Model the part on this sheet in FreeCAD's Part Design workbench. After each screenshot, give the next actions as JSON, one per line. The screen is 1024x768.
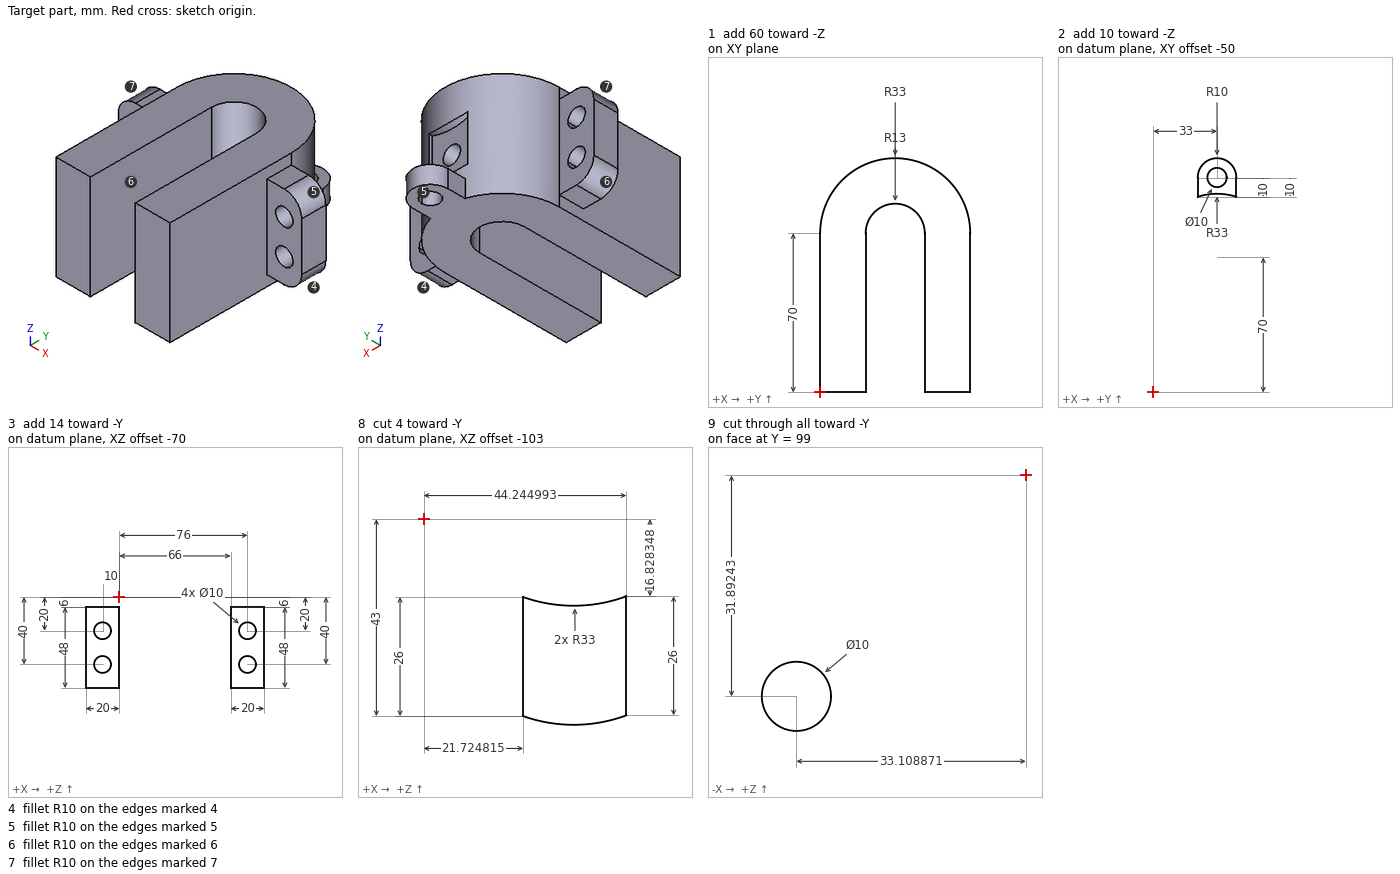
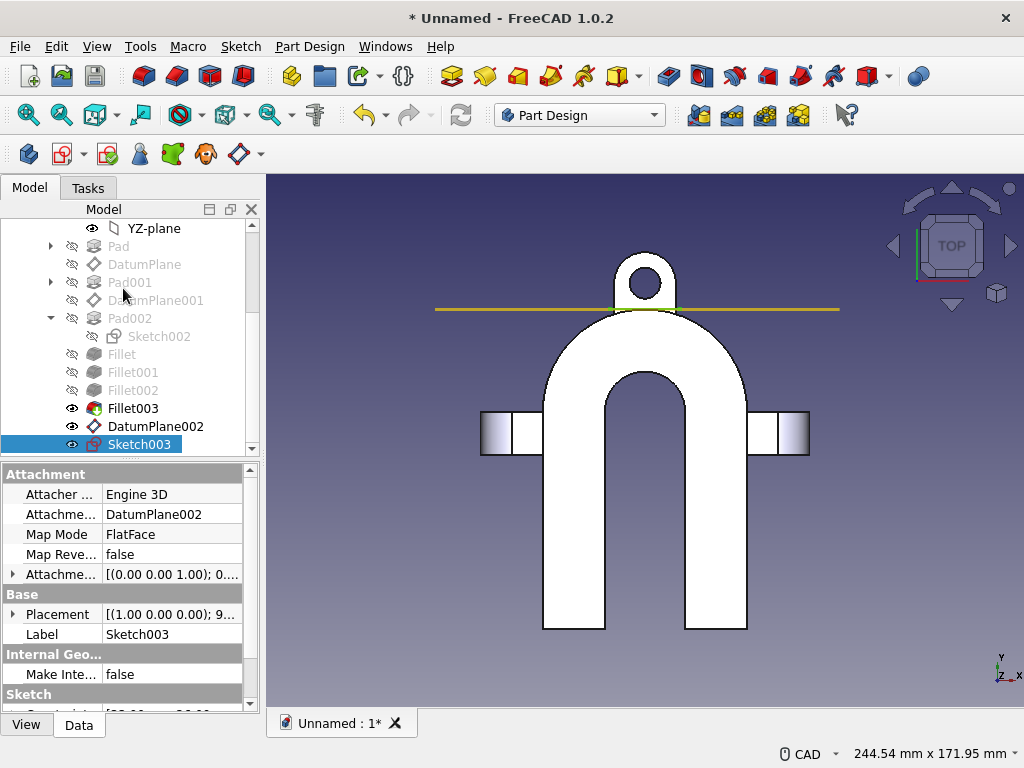
{"action": "left_click", "coordinate": [669, 76]}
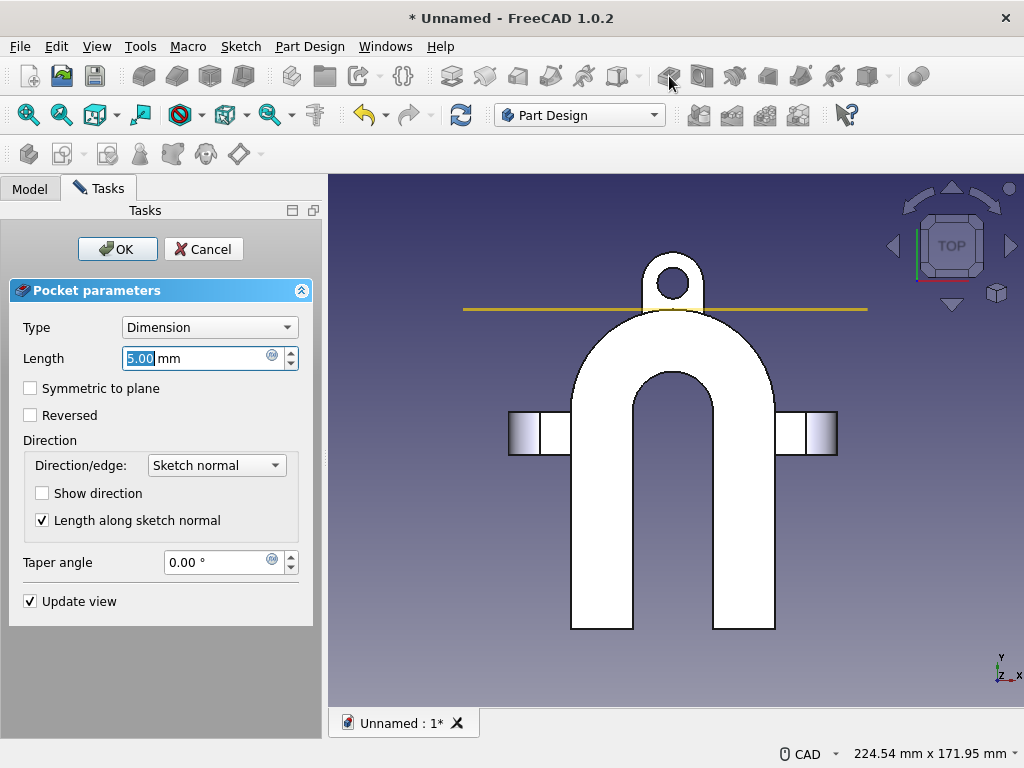
{"action": "type", "text": "4"}
{"action": "key", "text": "Tab"}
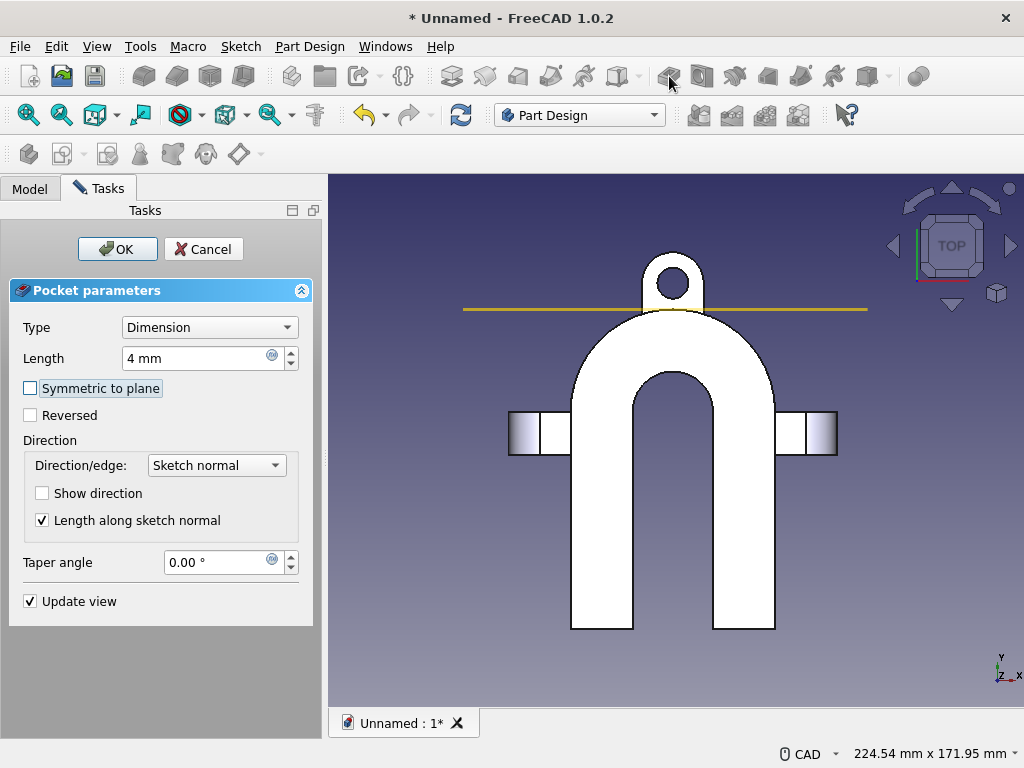
{"action": "left_click", "coordinate": [31, 415]}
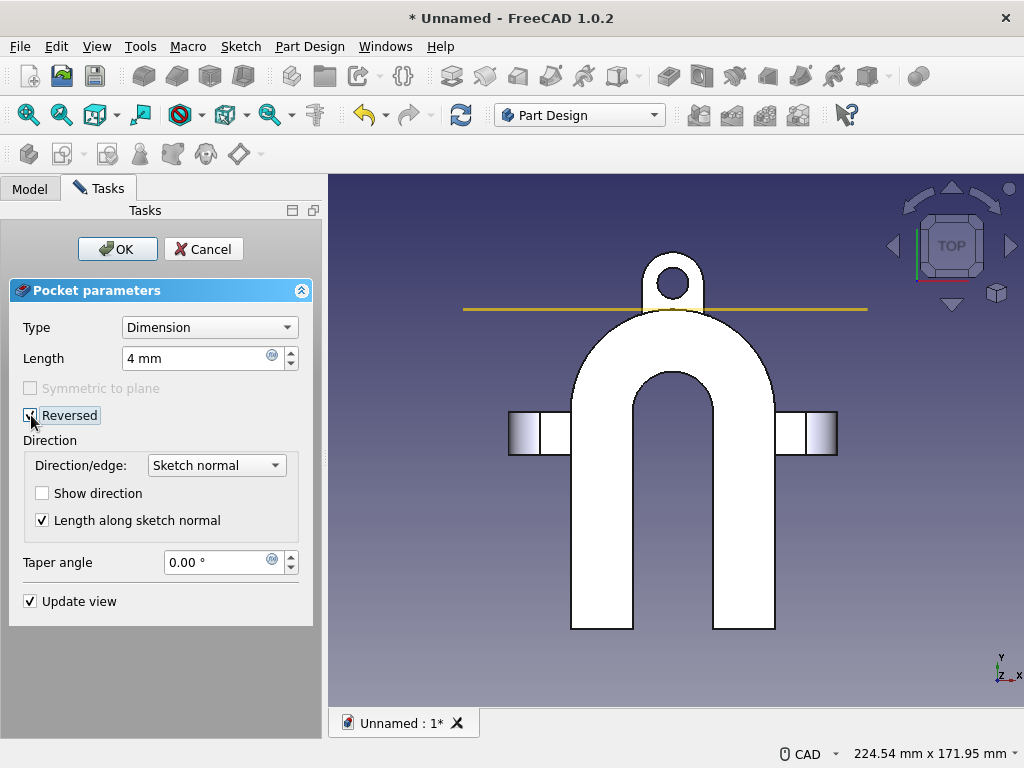
{"action": "left_click", "coordinate": [118, 249]}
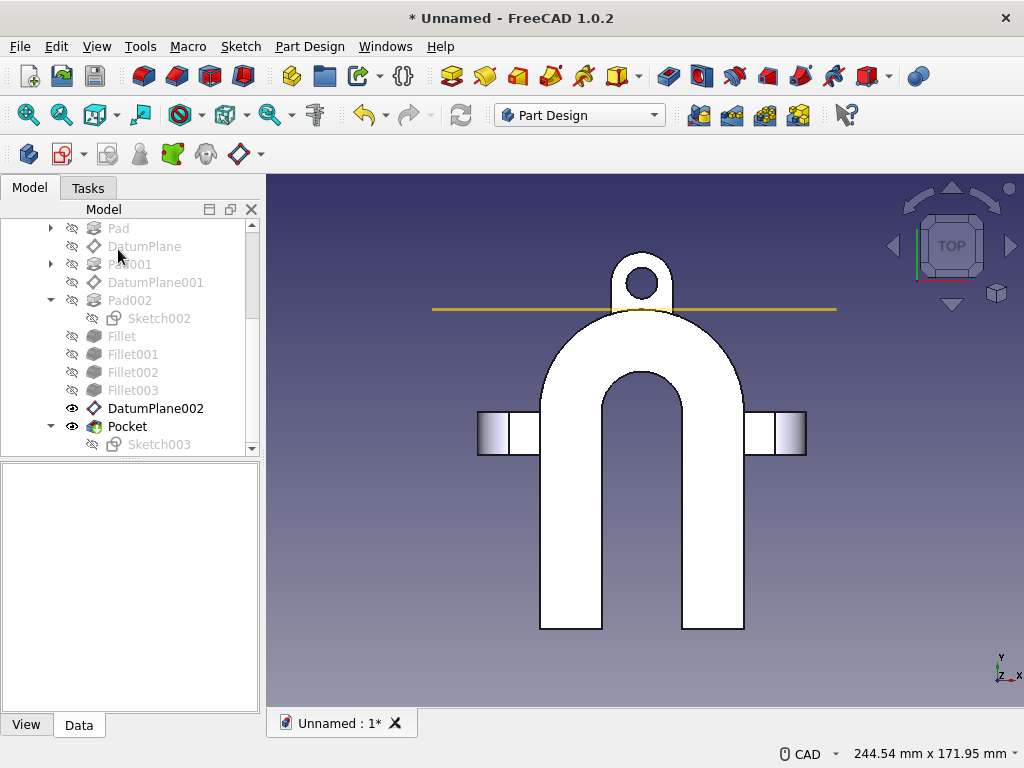
{"action": "left_click", "coordinate": [117, 408]}
{"action": "key", "text": "space"}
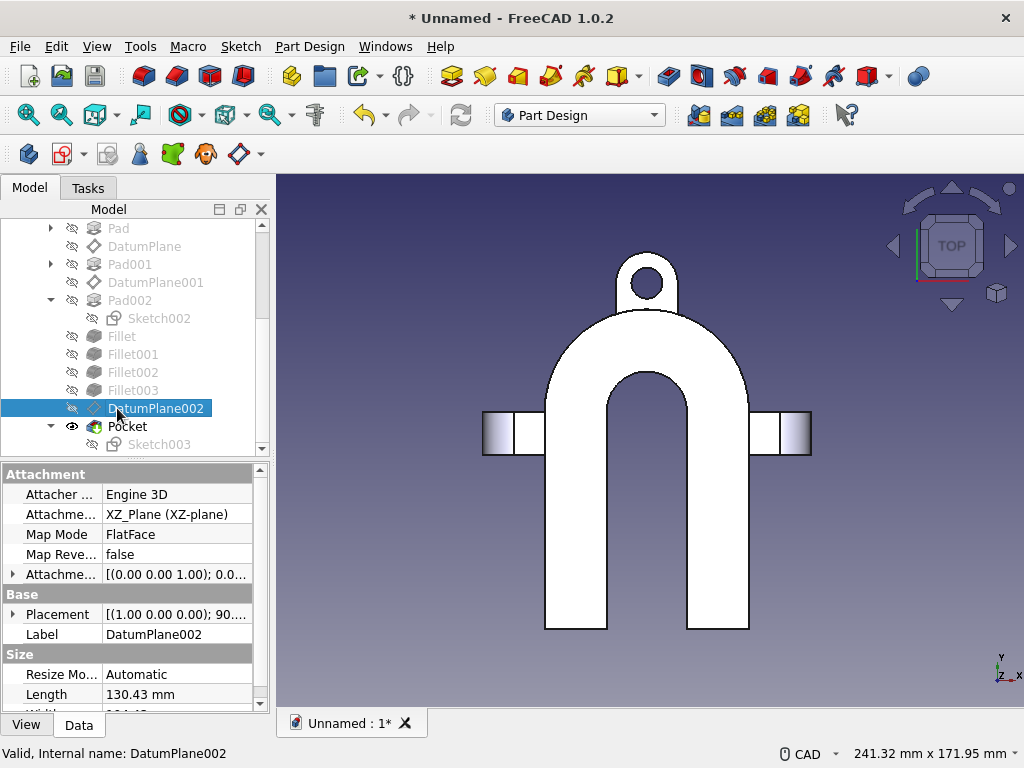
{"action": "key", "text": "4"}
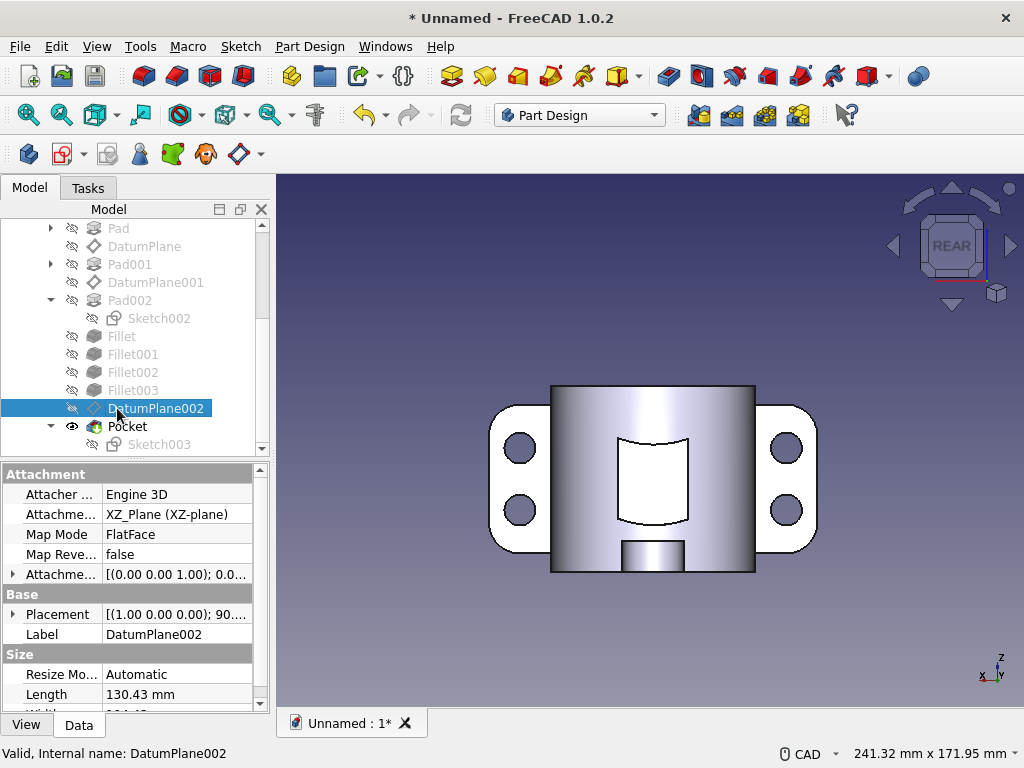
{"action": "left_click", "coordinate": [29, 116]}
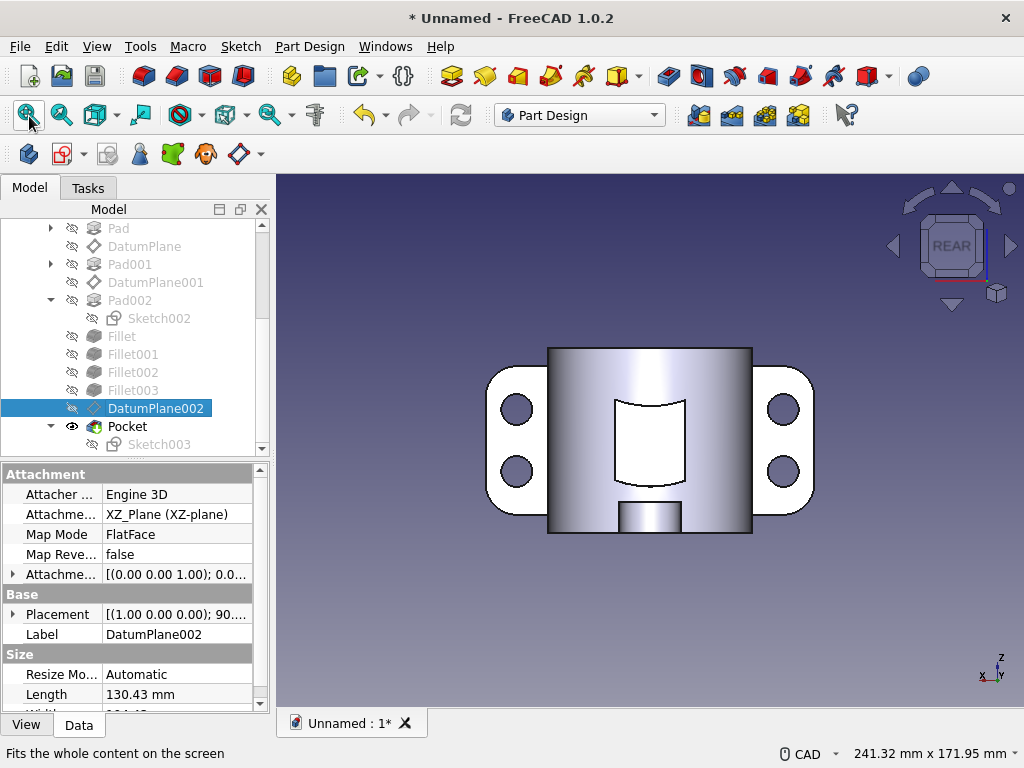
{"action": "left_click", "coordinate": [650, 442]}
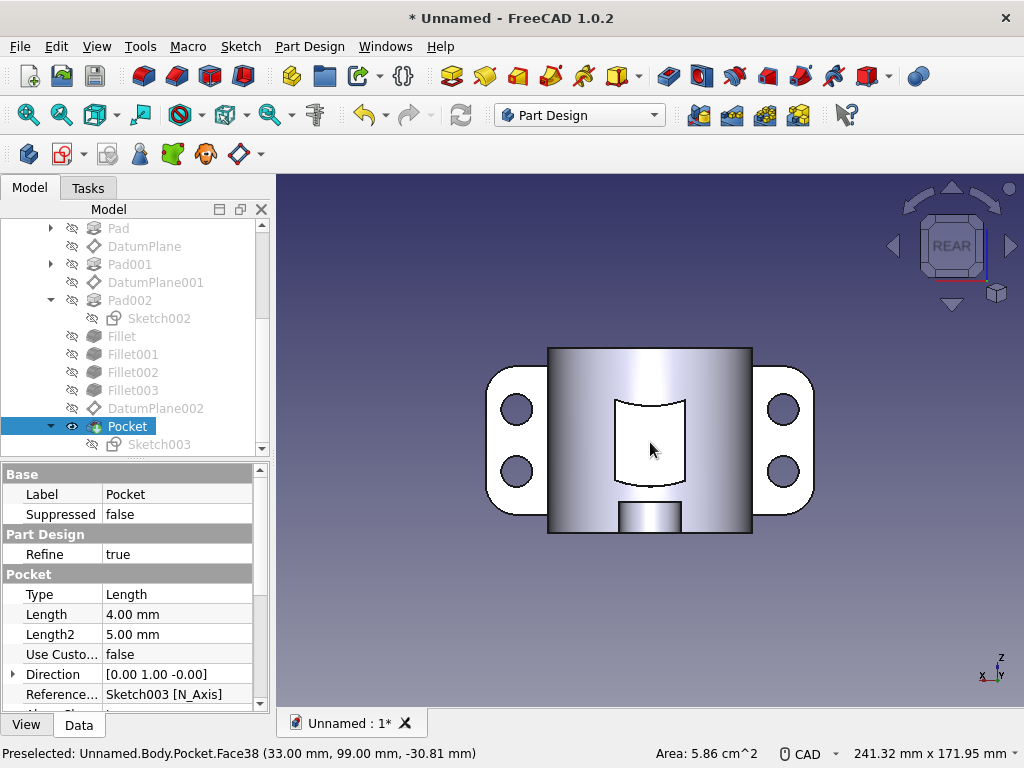
{"action": "left_click", "coordinate": [62, 154]}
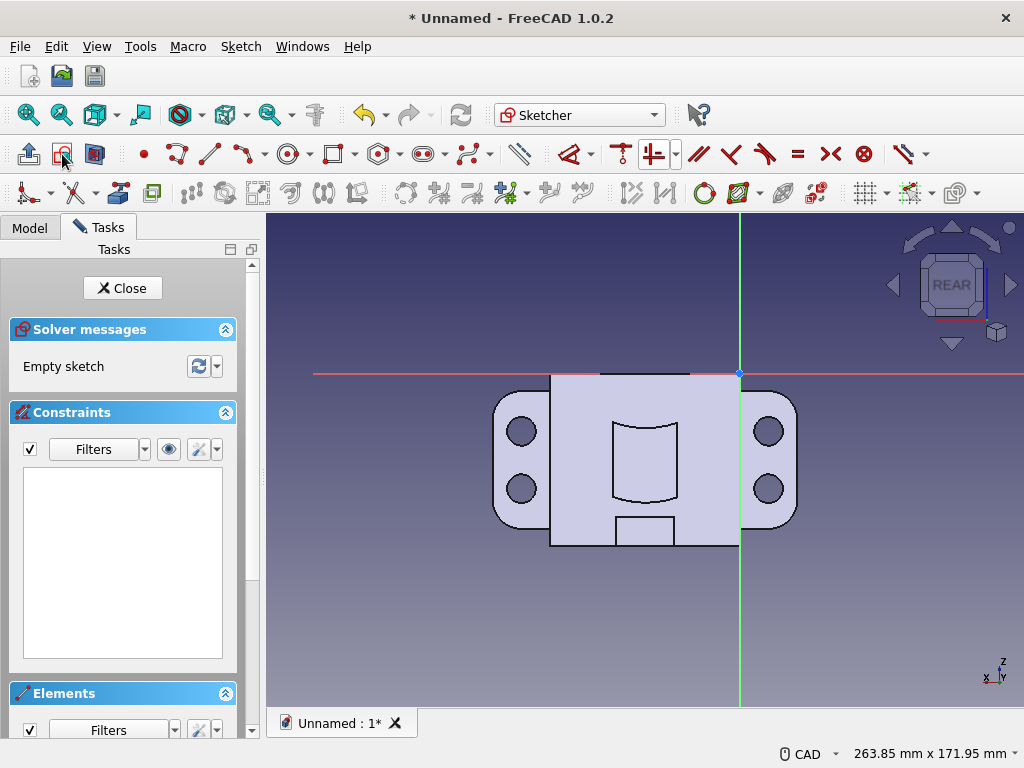
{"action": "left_click", "coordinate": [95, 154]}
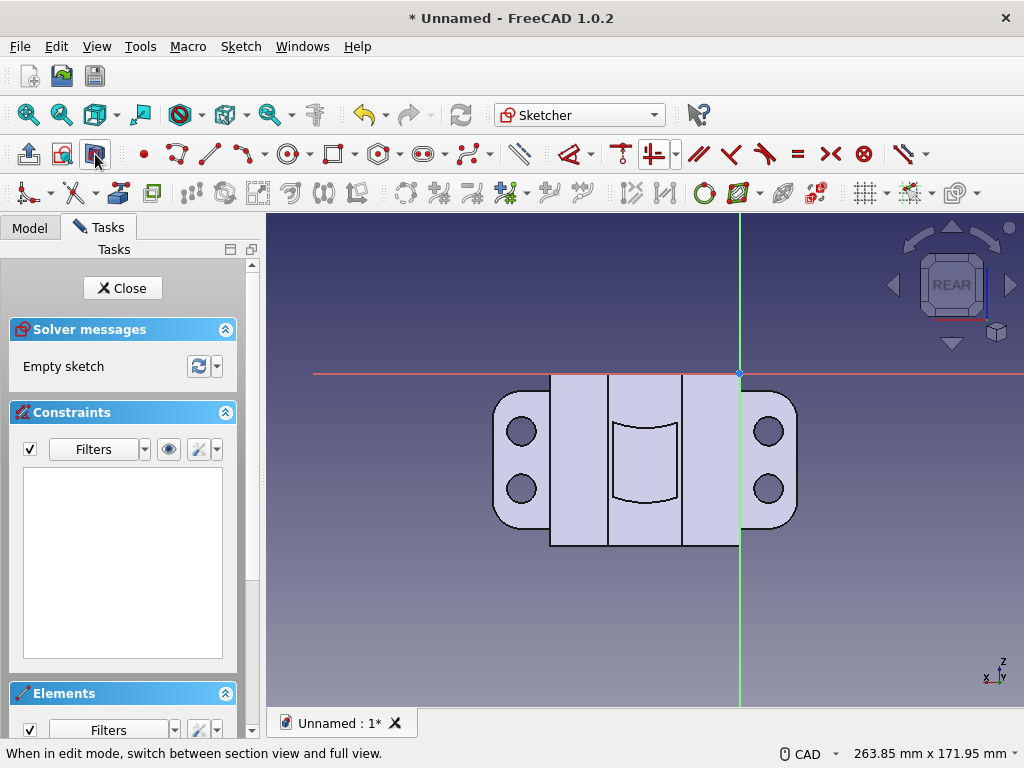
{"action": "scroll", "coordinate": [651, 466], "scroll_direction": "up", "scroll_amount": 12}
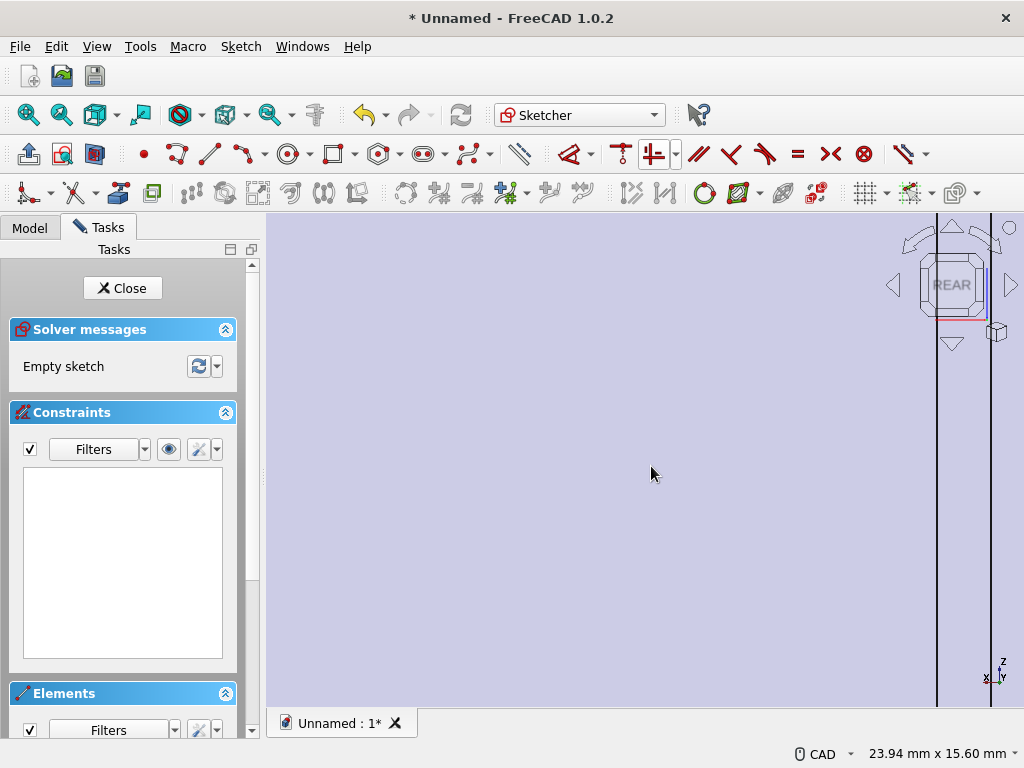
{"action": "key", "text": "g c"}